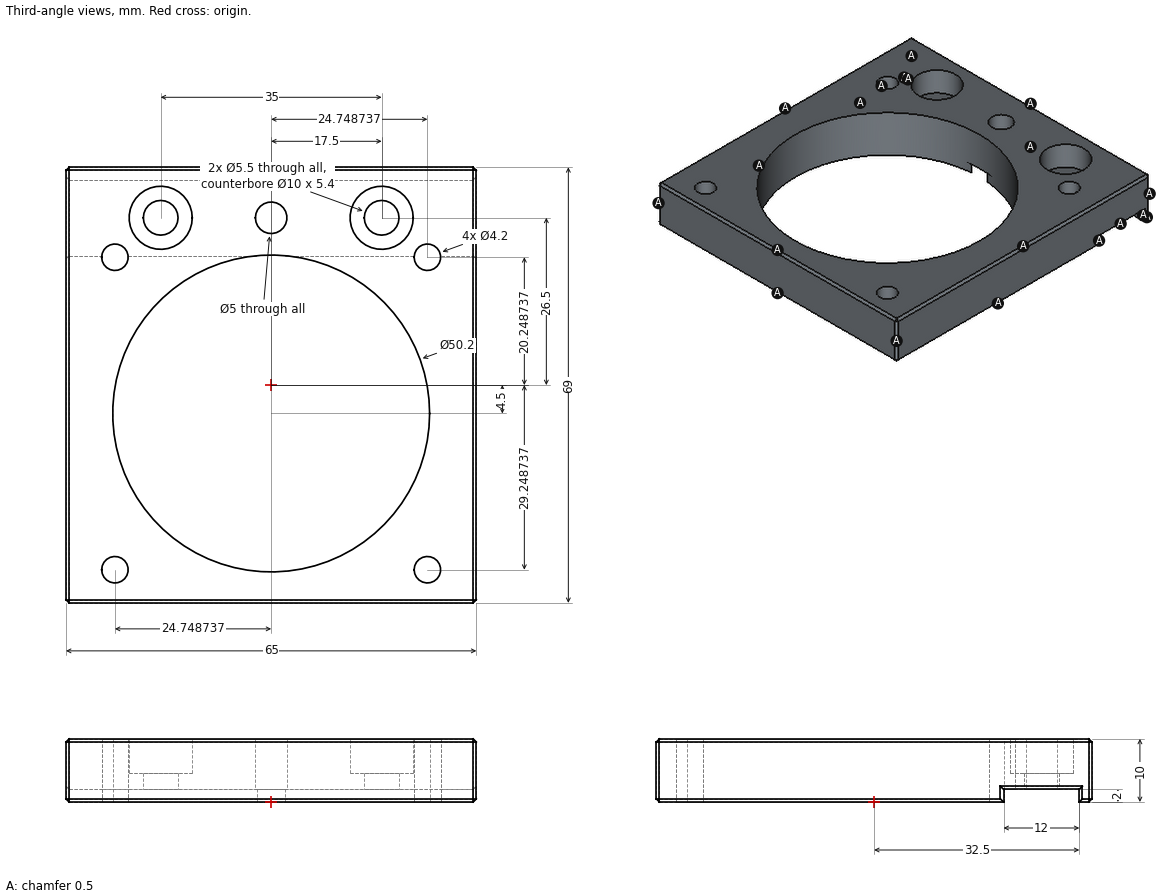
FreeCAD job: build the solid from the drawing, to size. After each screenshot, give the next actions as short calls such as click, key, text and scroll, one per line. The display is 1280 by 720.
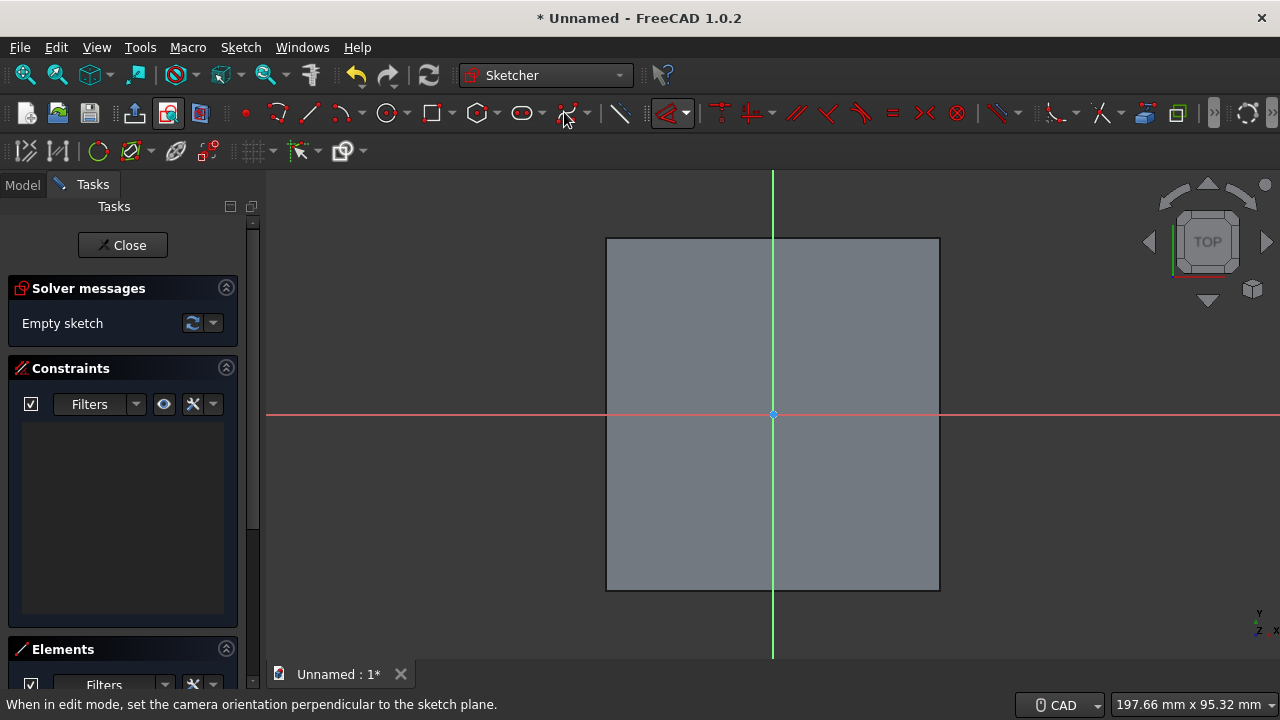
click(388, 114)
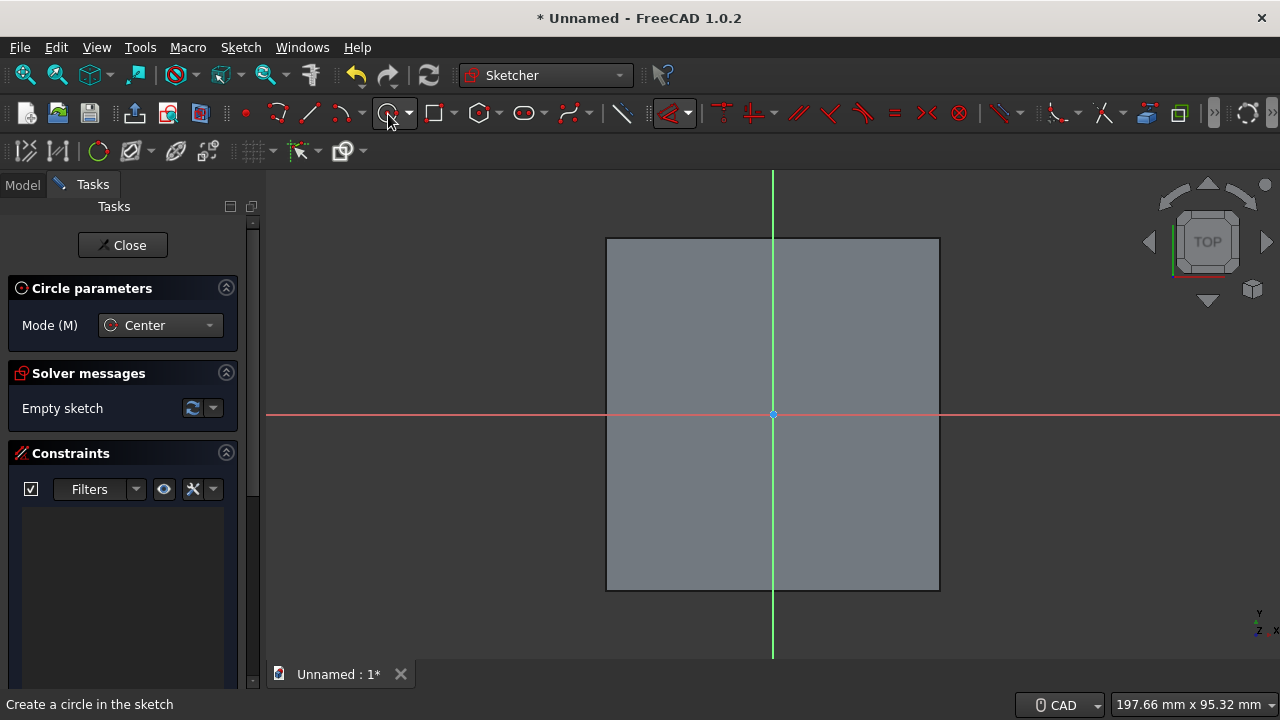
click(773, 438)
click(864, 347)
key(Escape)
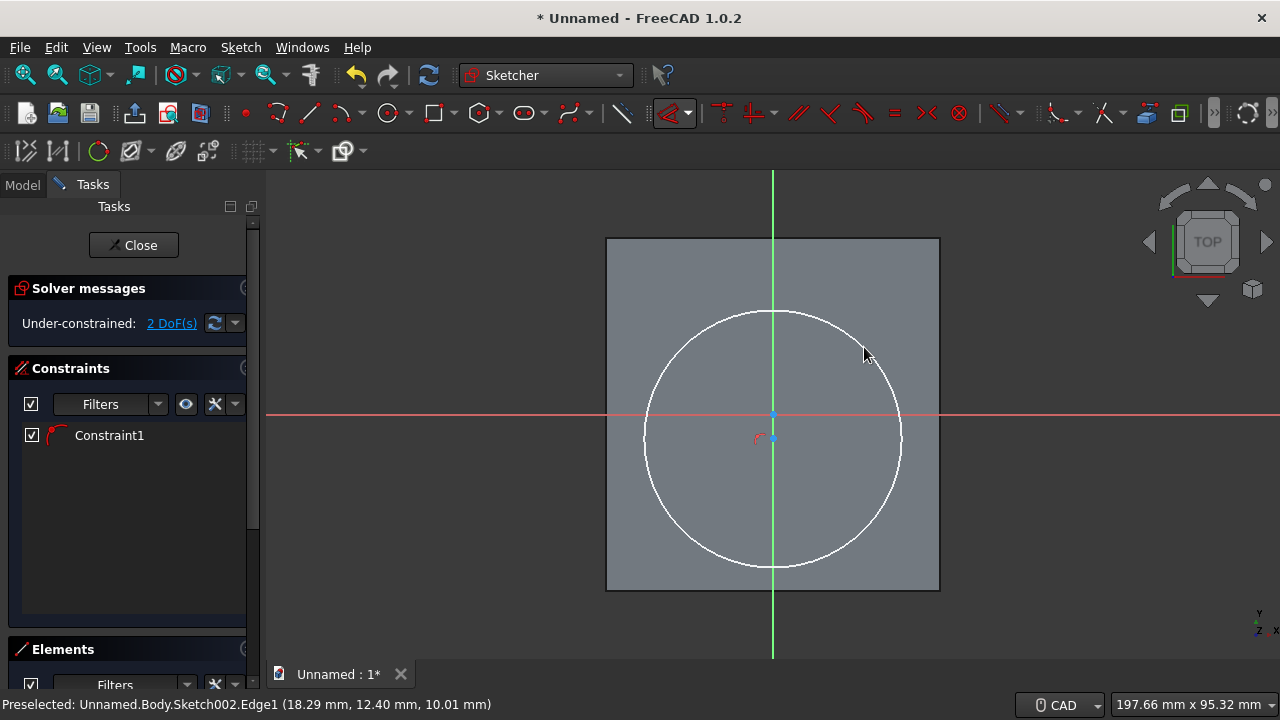
click(864, 348)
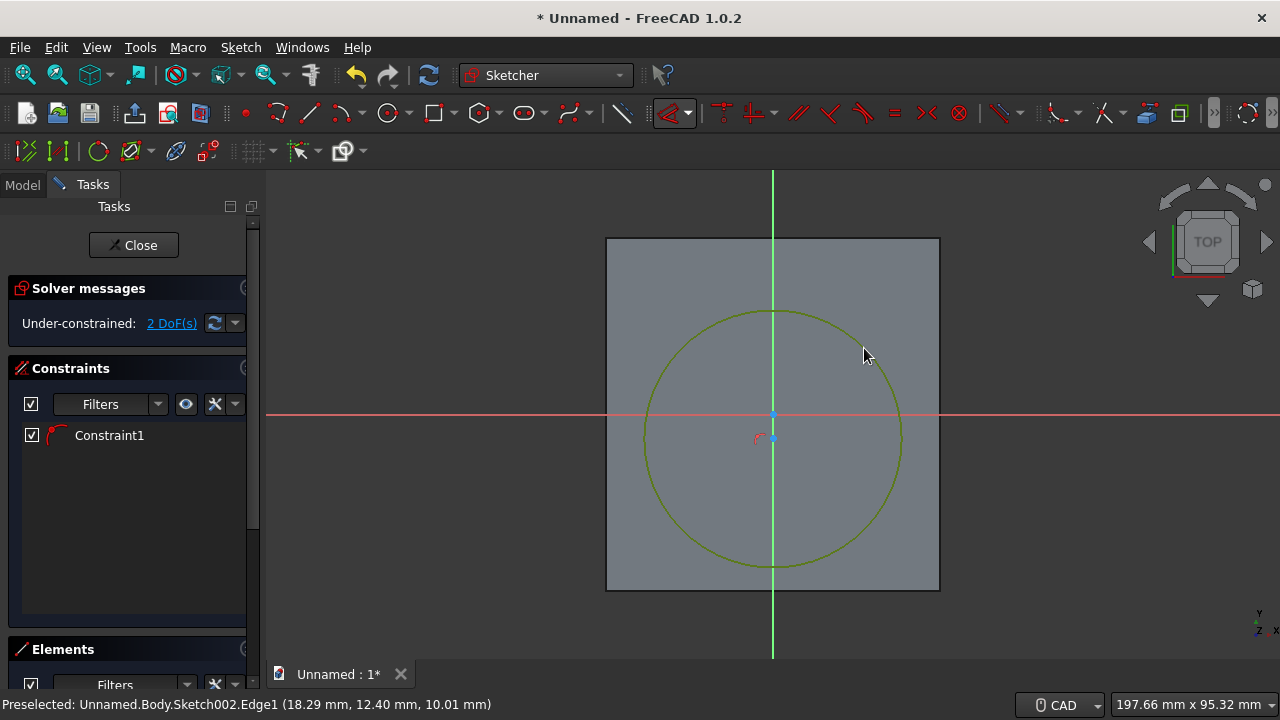
key(k)
key(o)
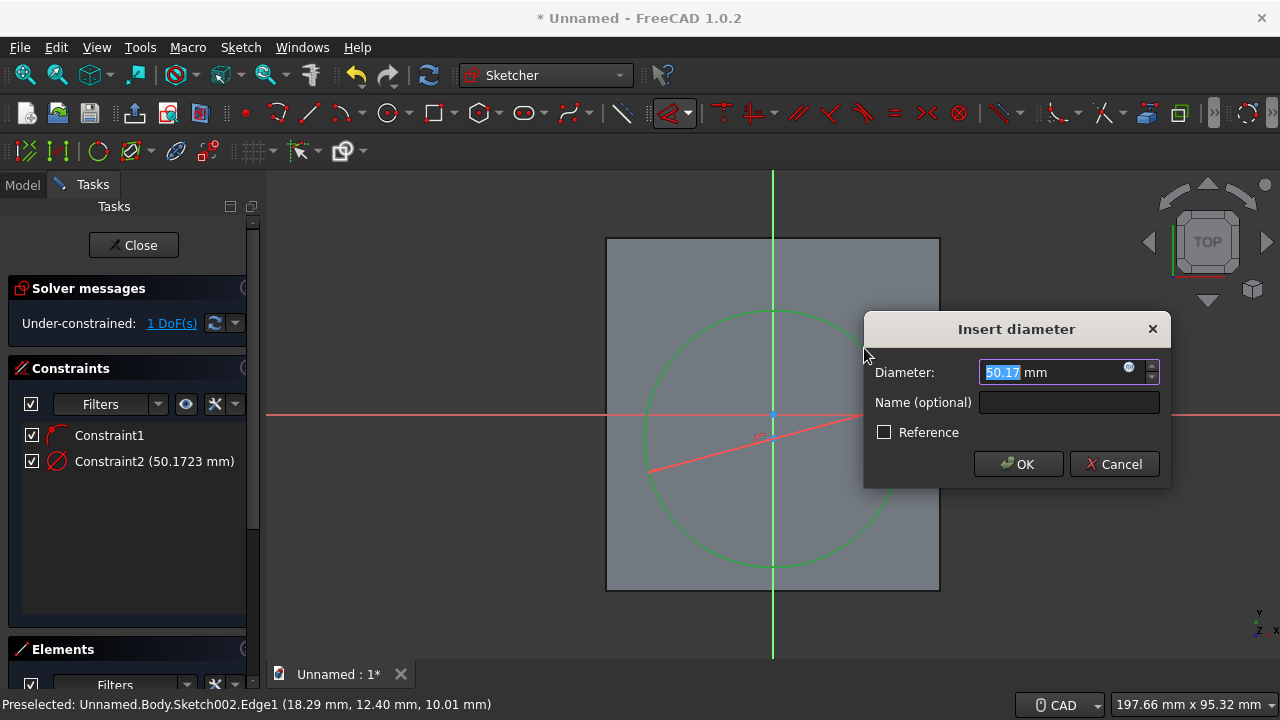
text(50.2)
key(Return)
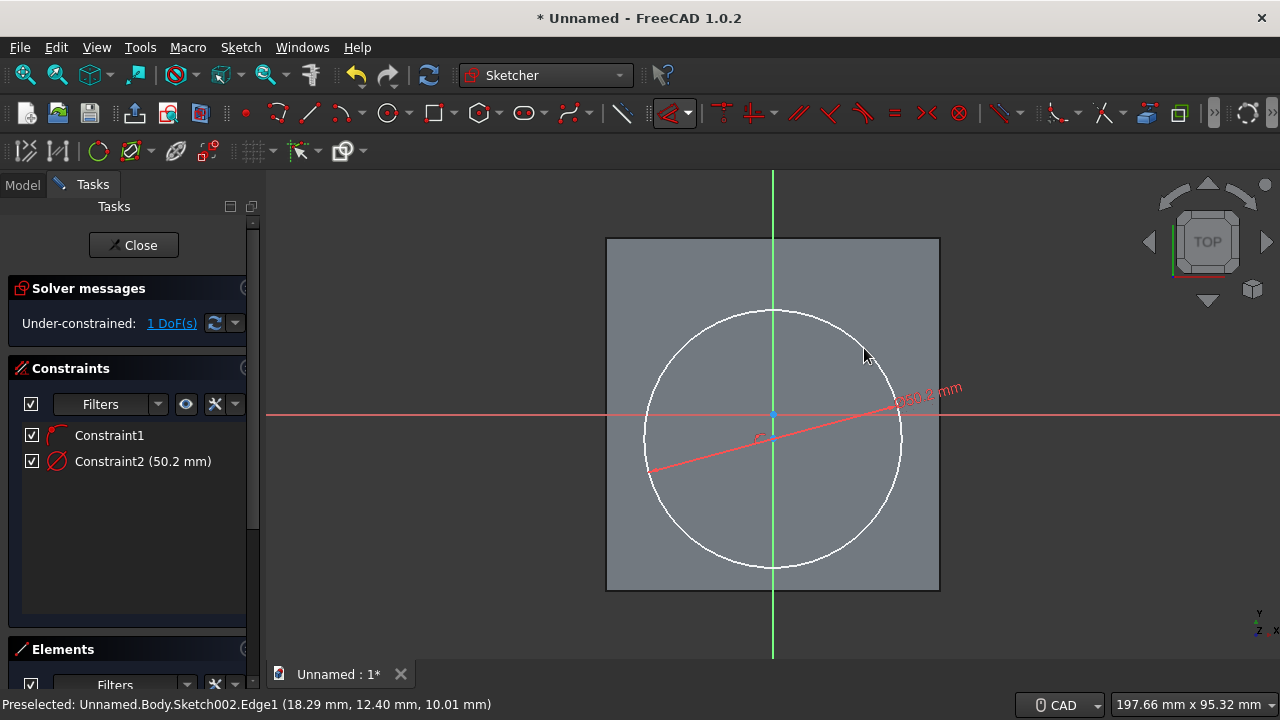
scroll(773, 439, up, 3)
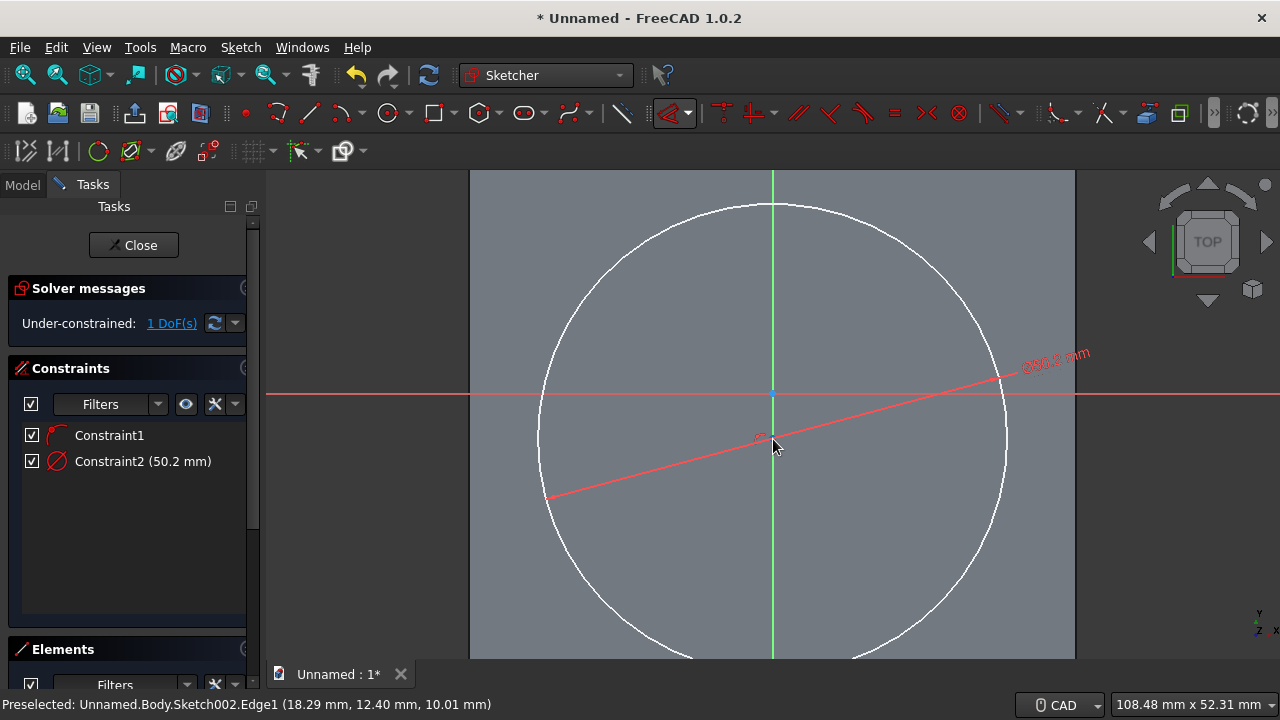
click(773, 439)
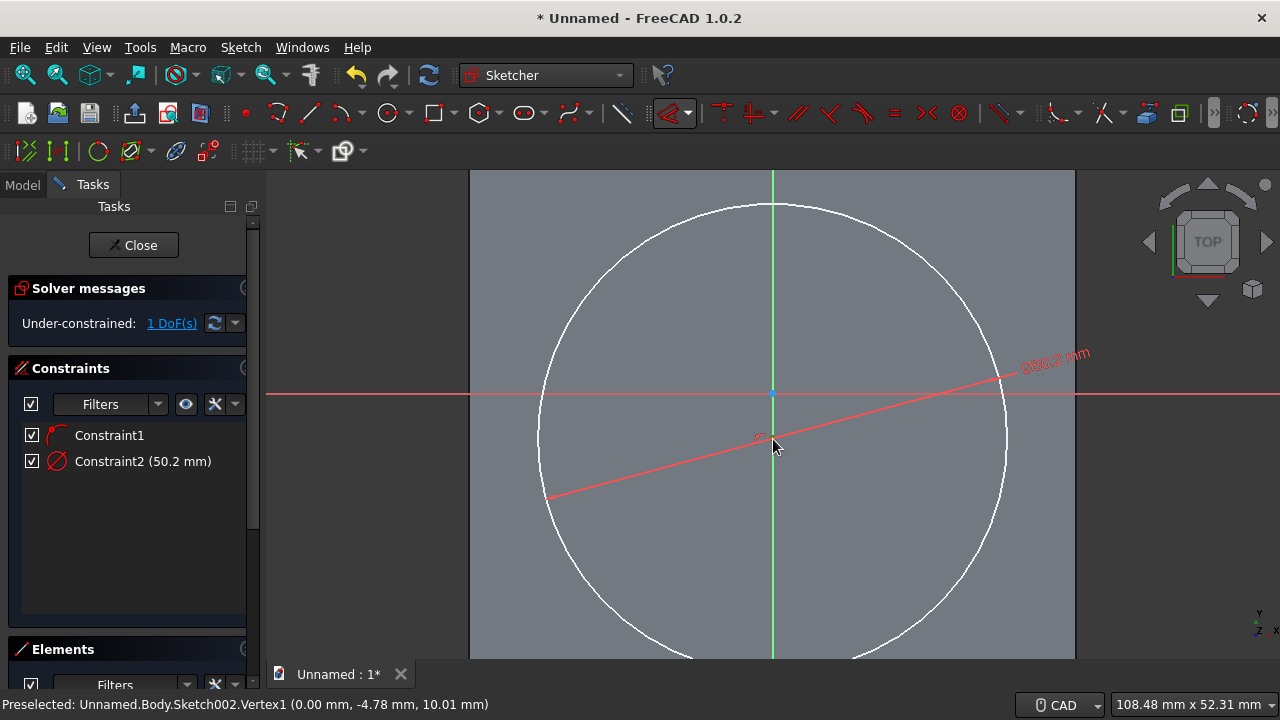
click(690, 114)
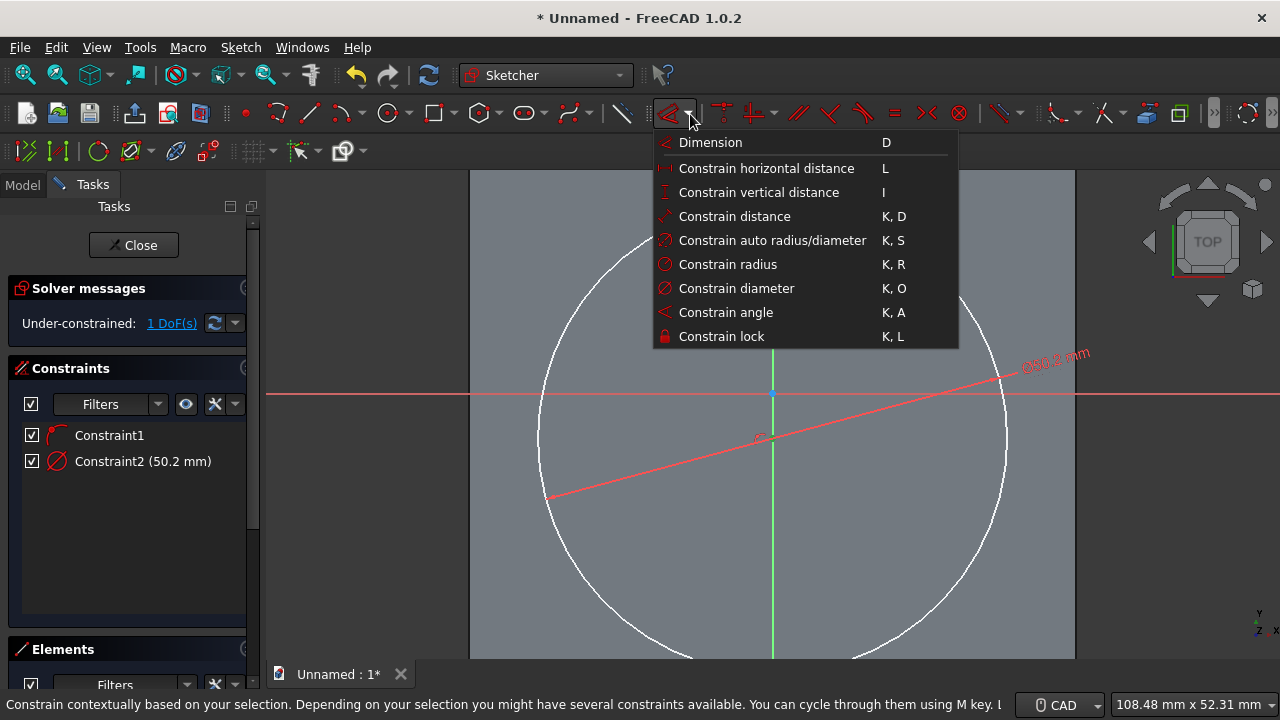
click(806, 192)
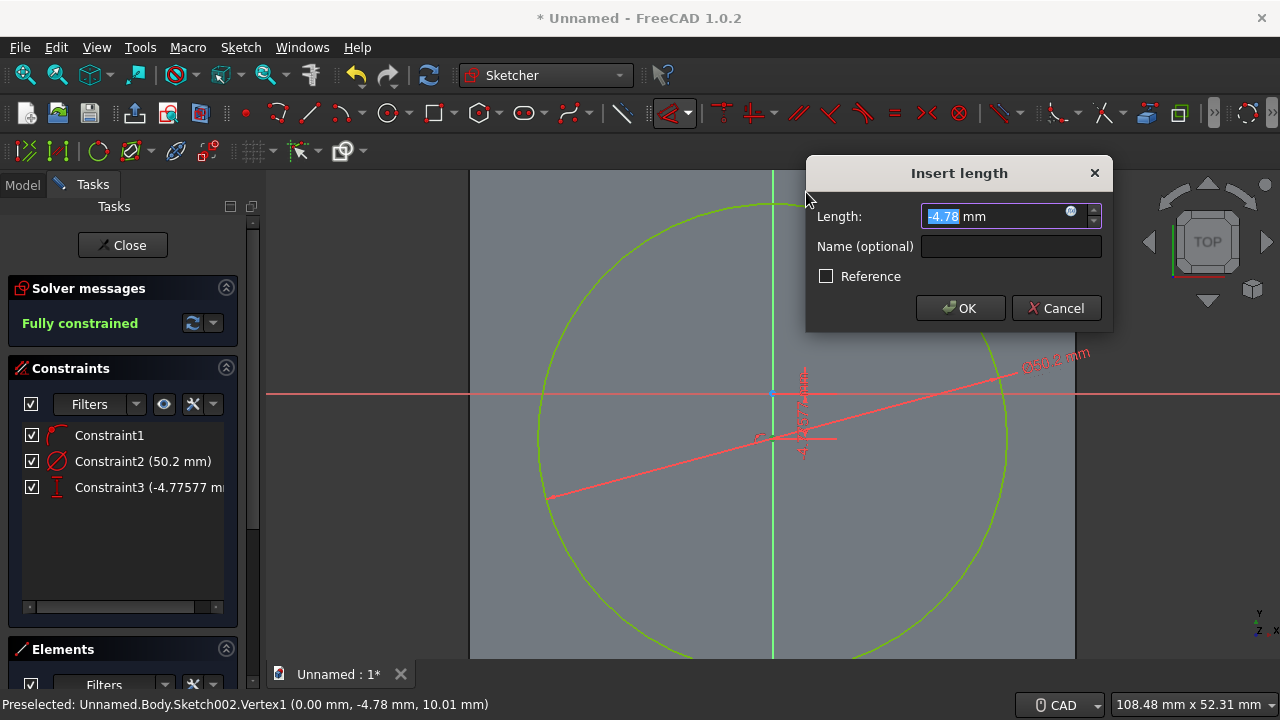
text(-4.5)
key(Return)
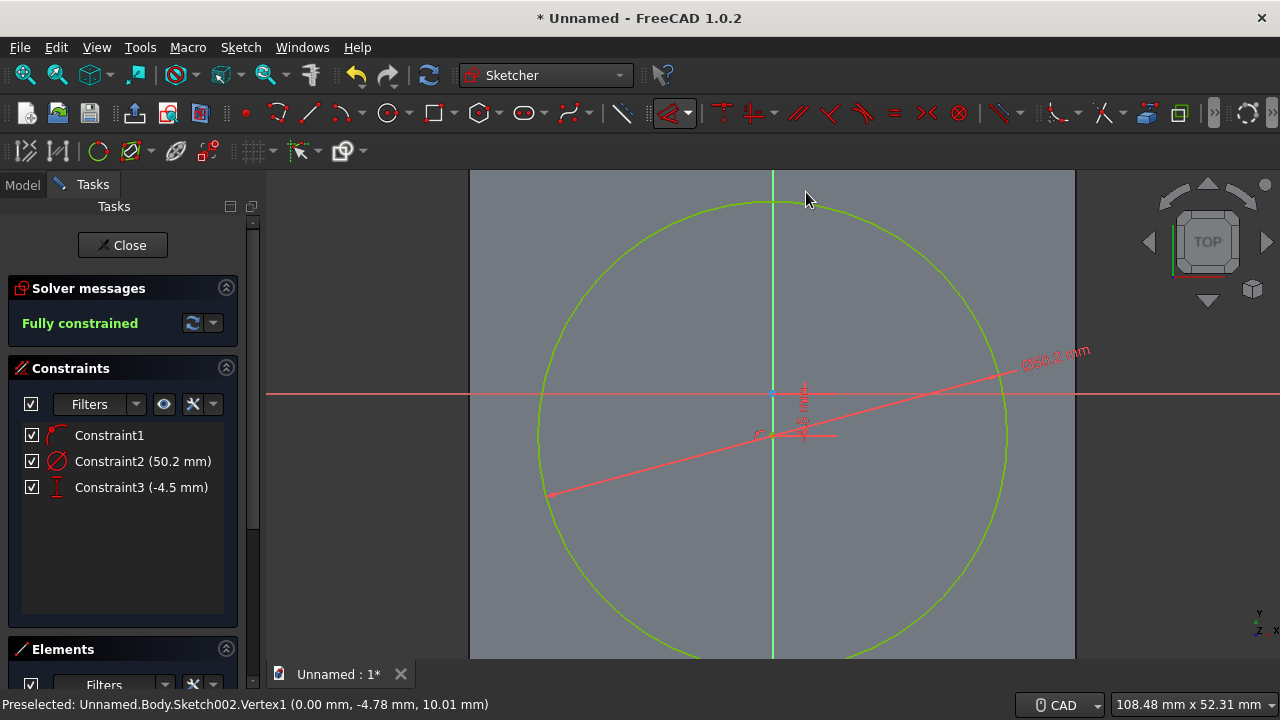
click(123, 245)